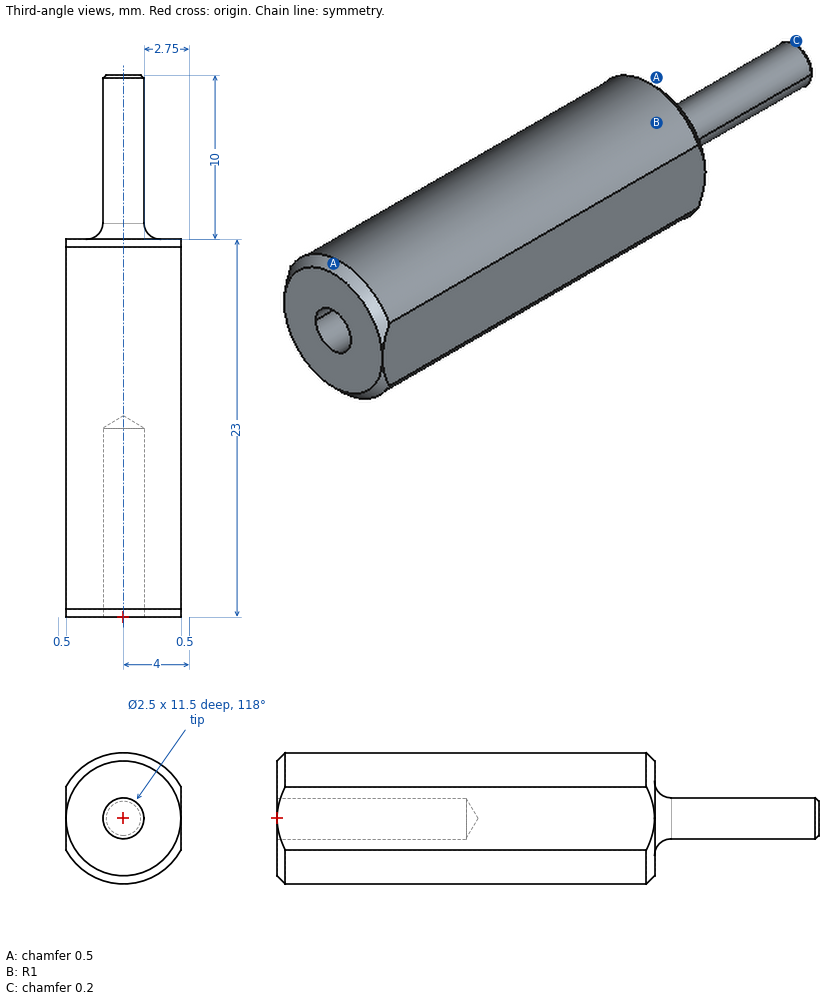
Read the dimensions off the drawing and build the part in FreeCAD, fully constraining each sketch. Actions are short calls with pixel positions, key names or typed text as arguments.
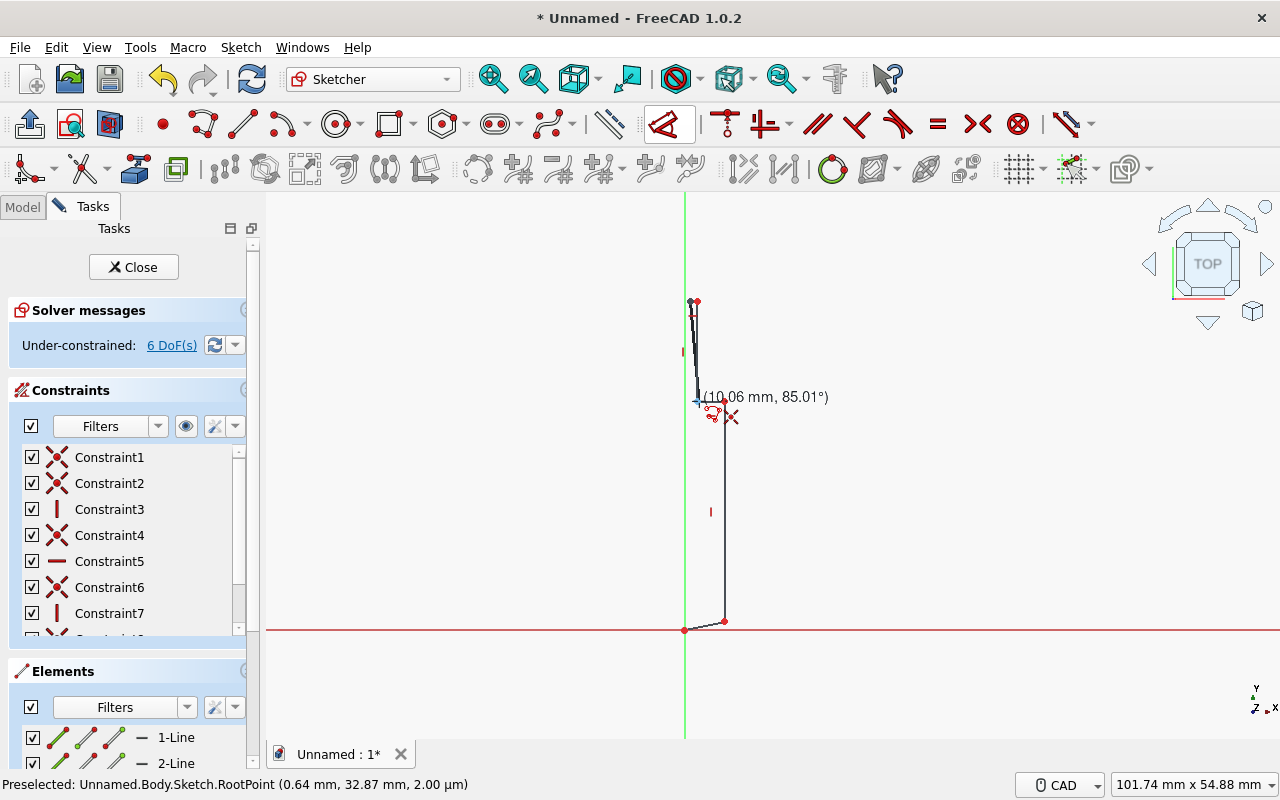
click(685, 630)
key(Escape)
key(Escape)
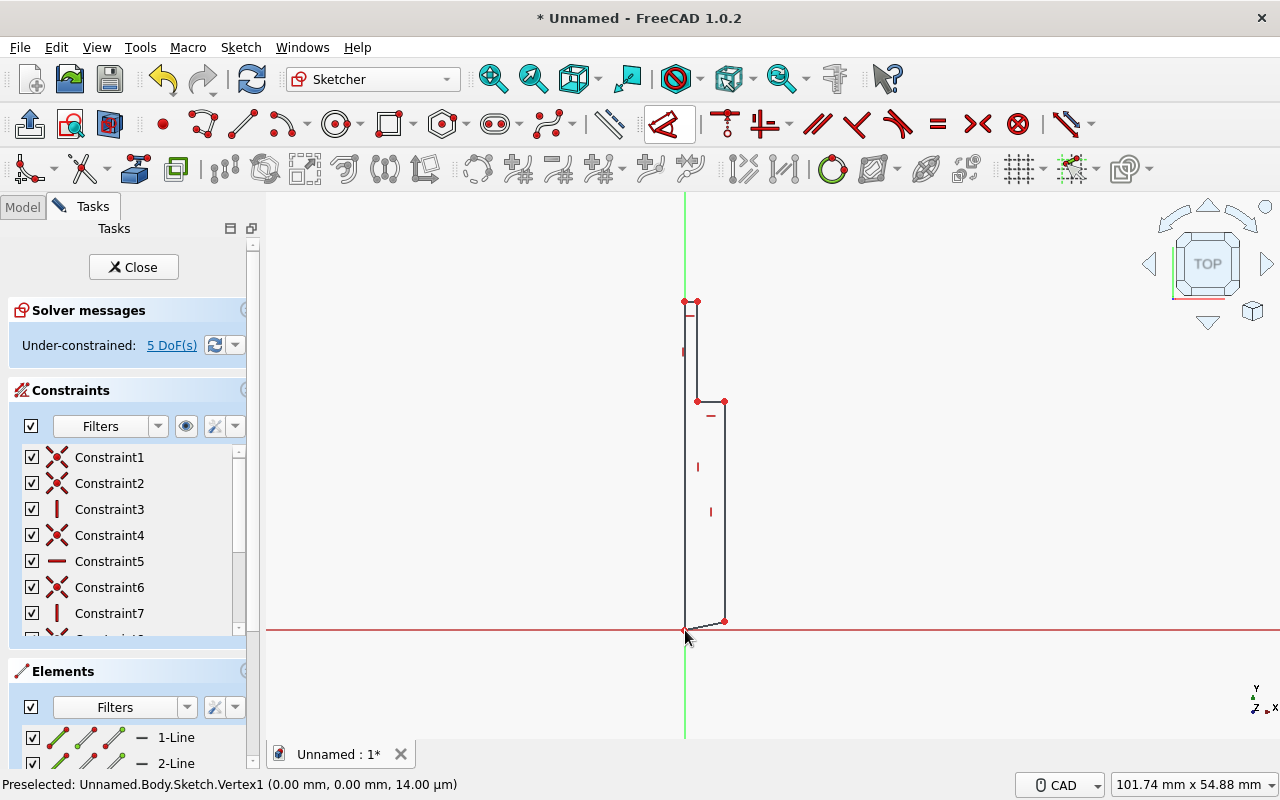
click(697, 628)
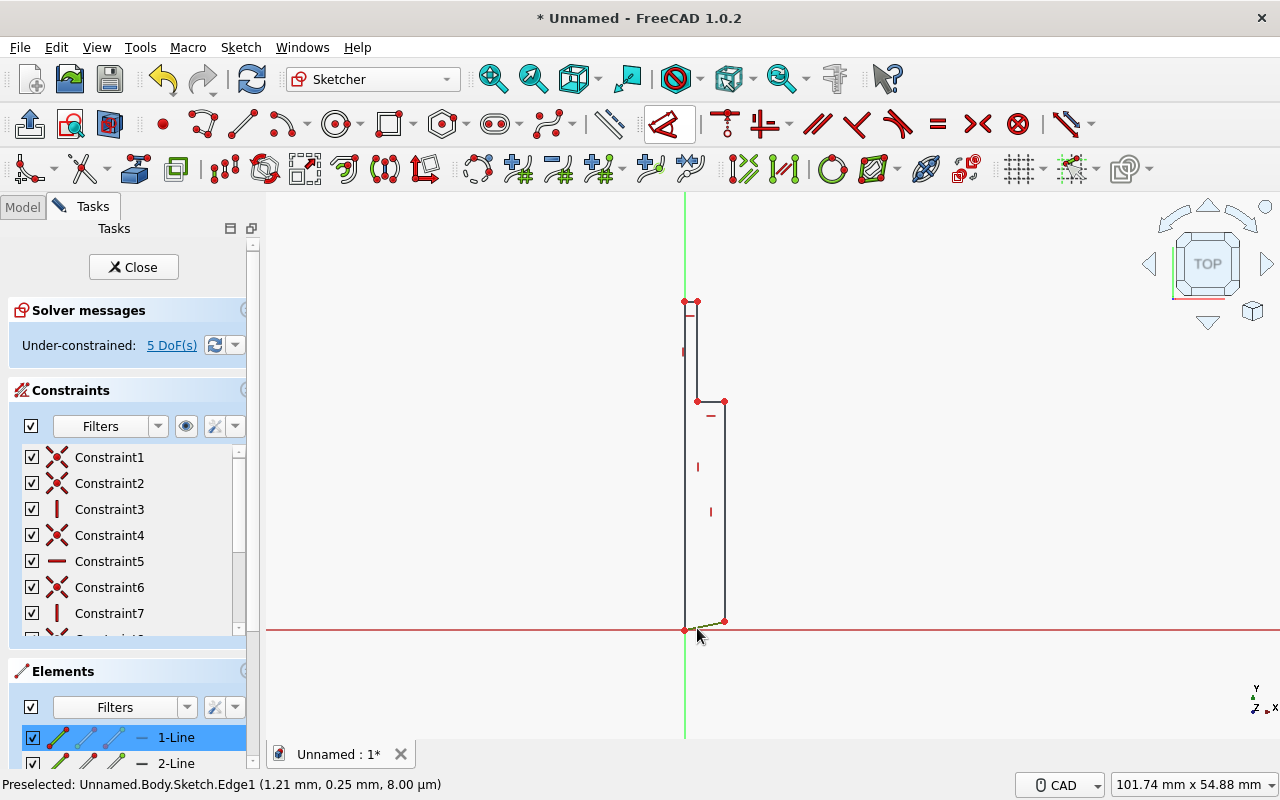
key(h)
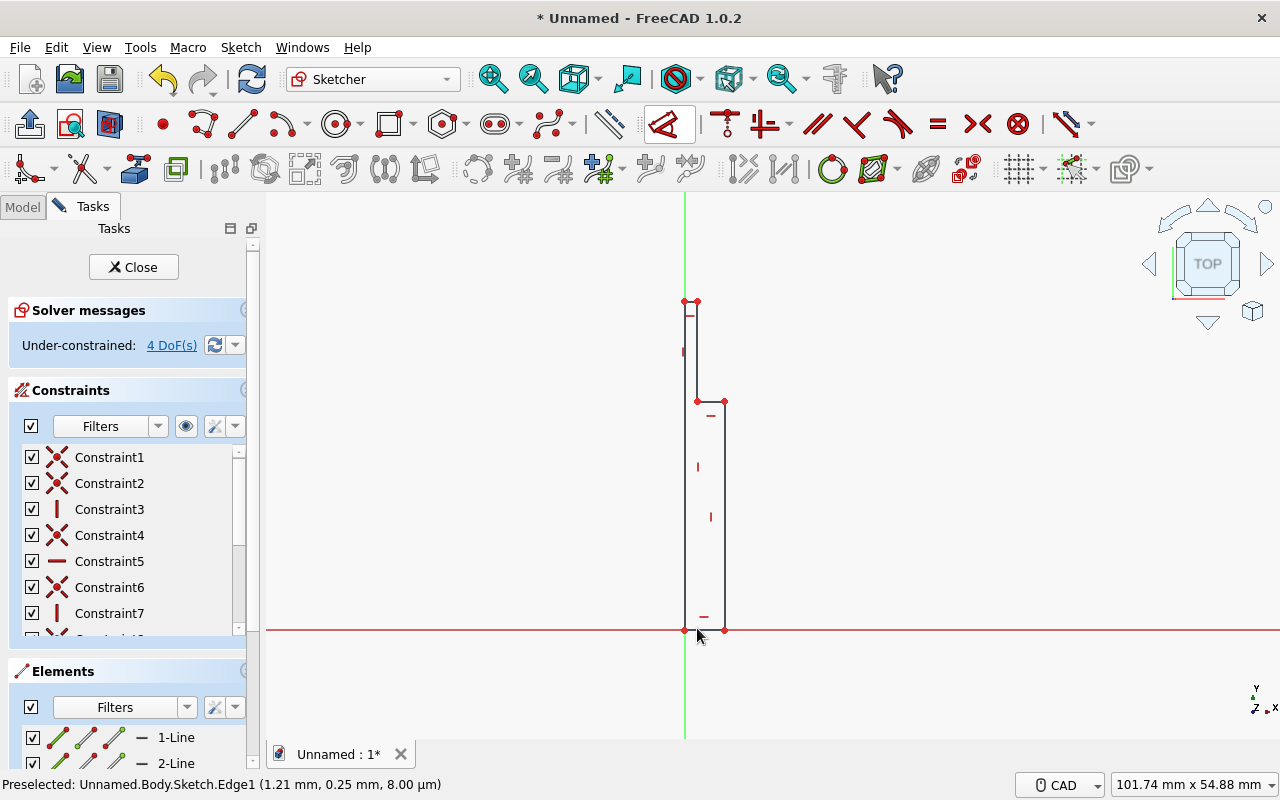
click(697, 630)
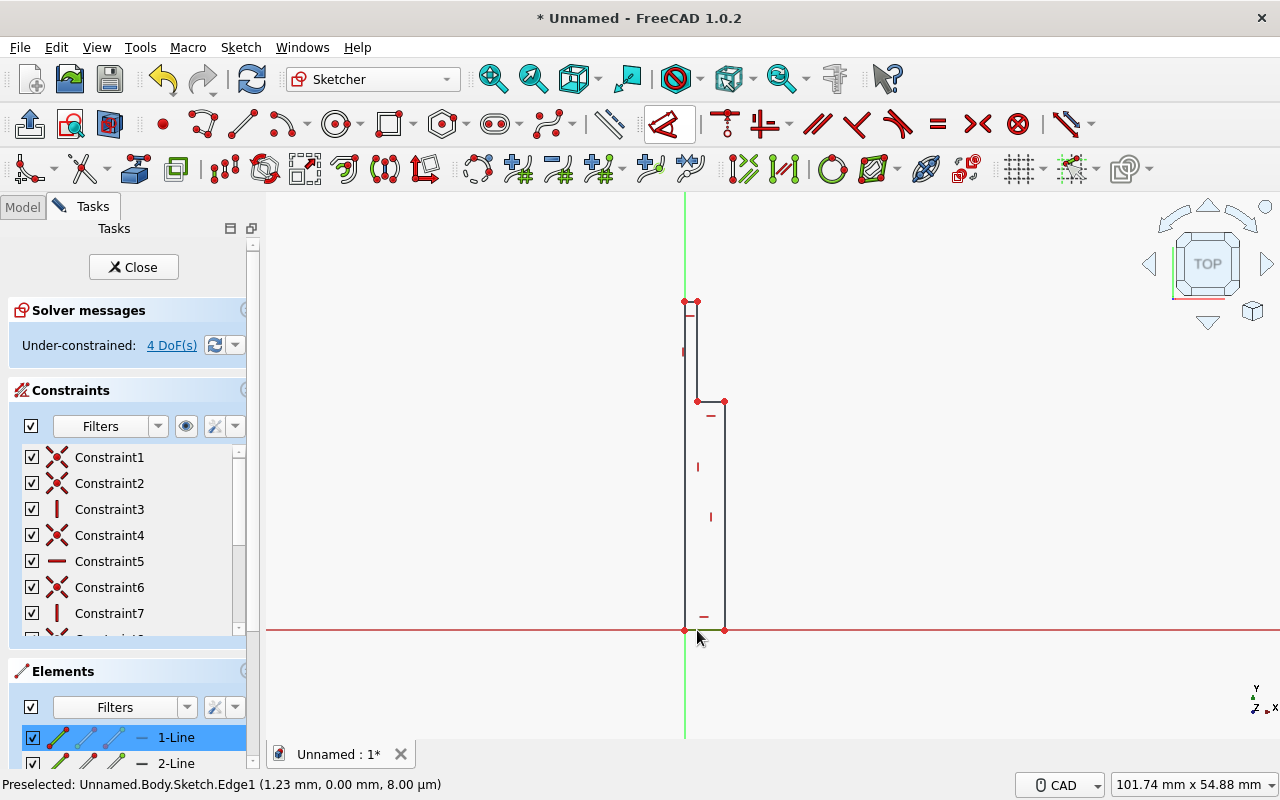
key(l)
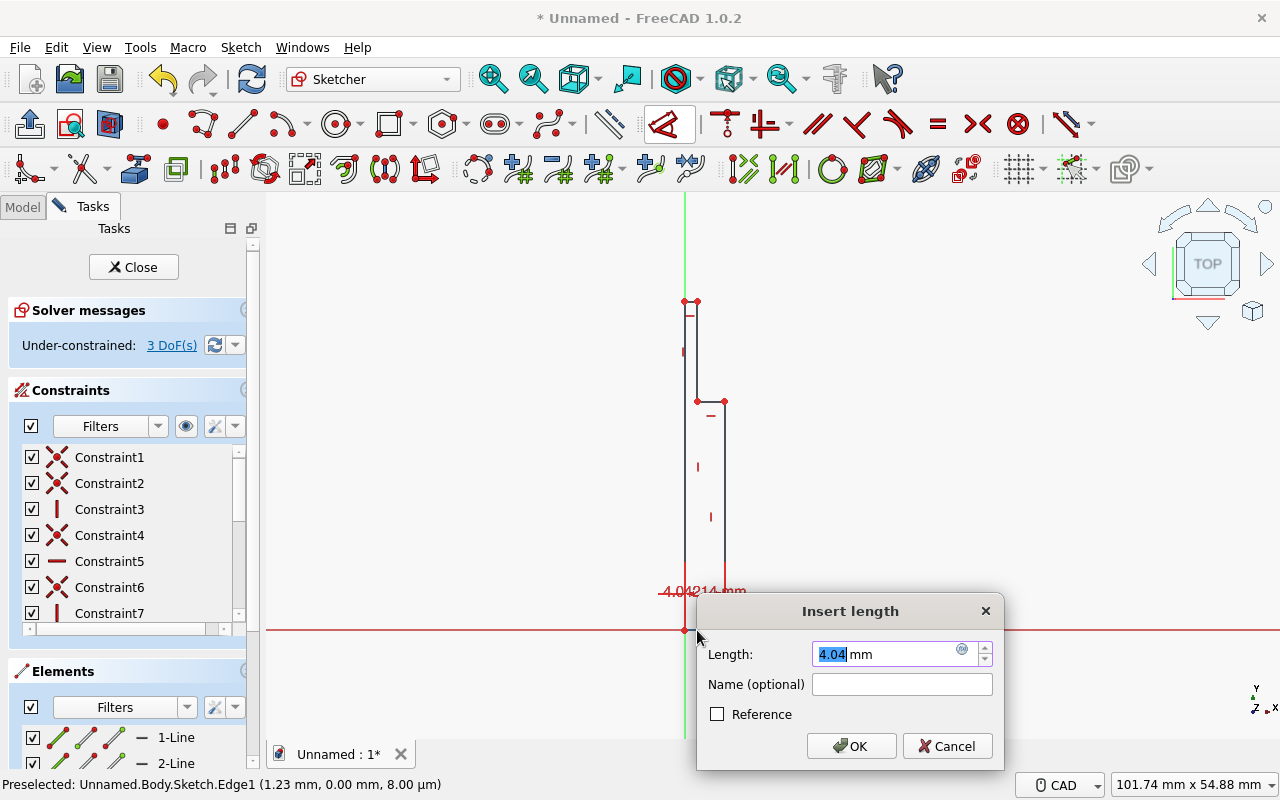
text(4)
key(Return)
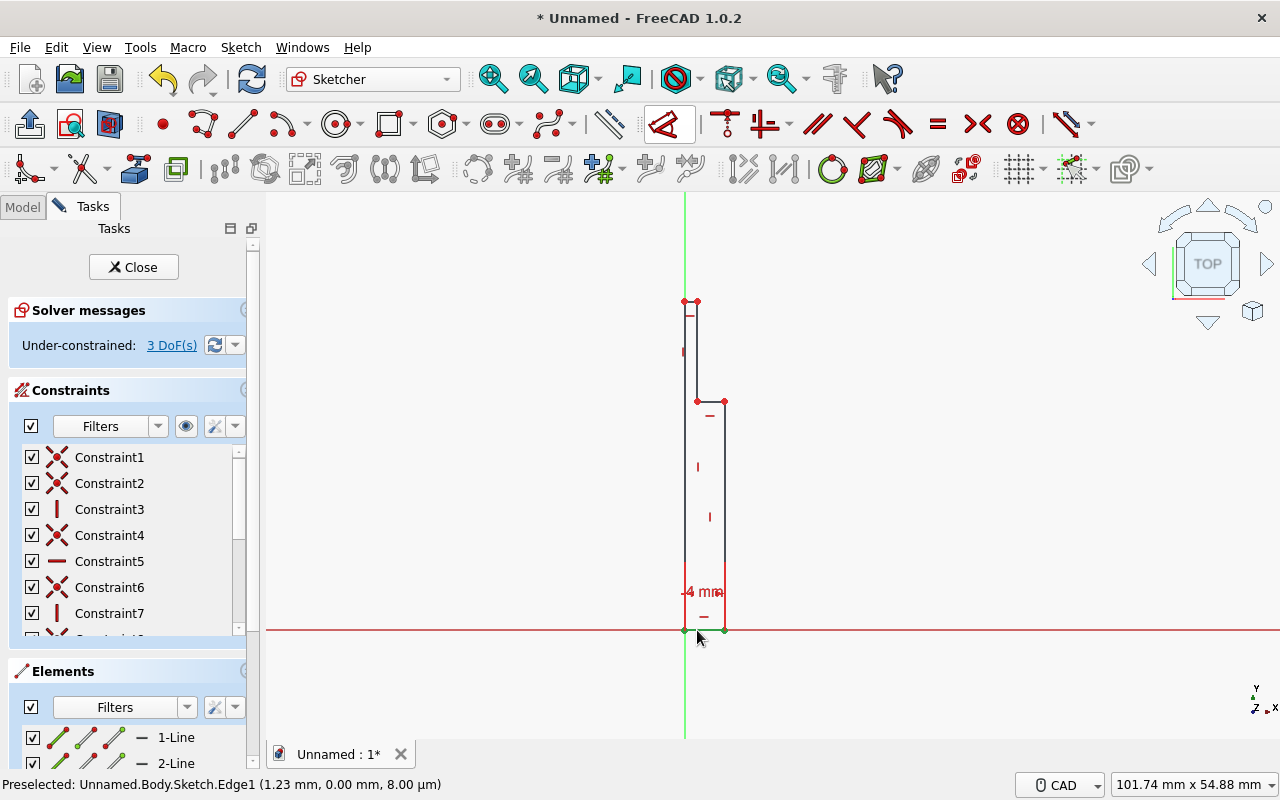
click(725, 562)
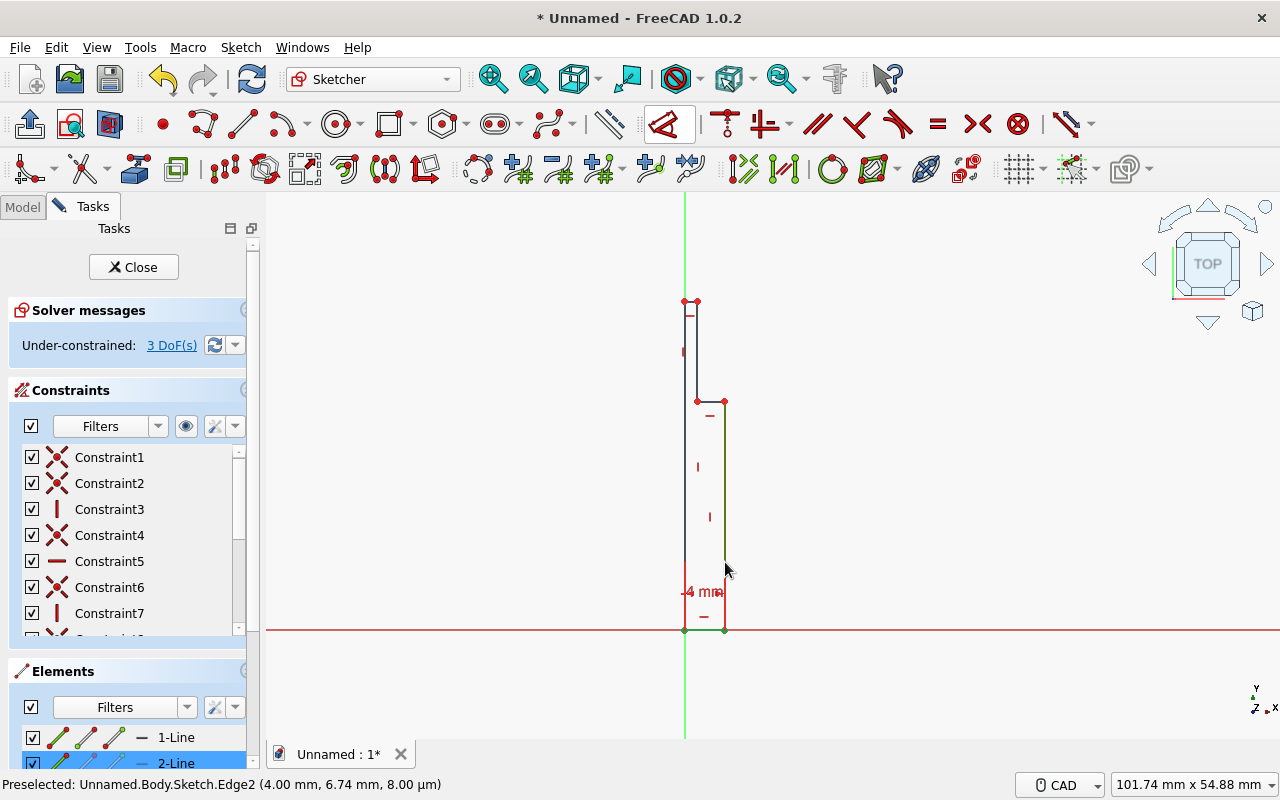
key(i)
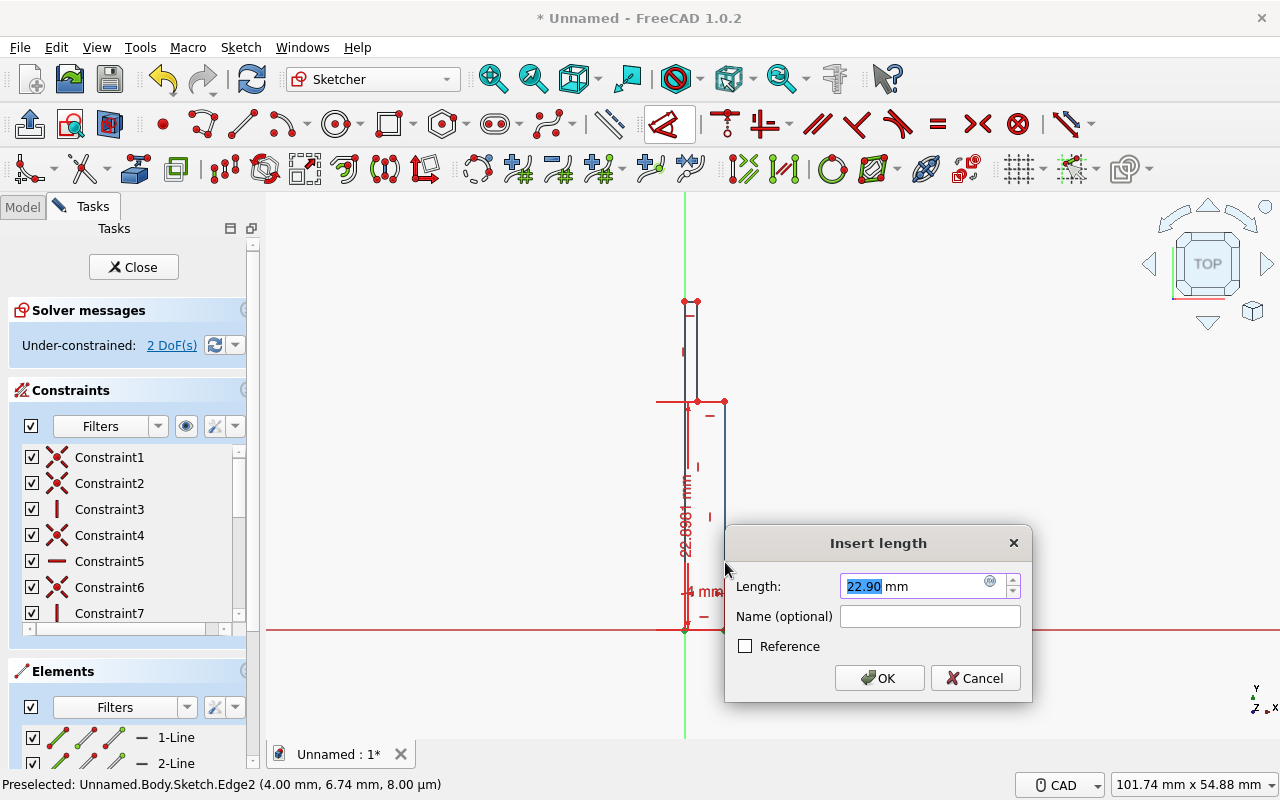
text(23)
key(Return)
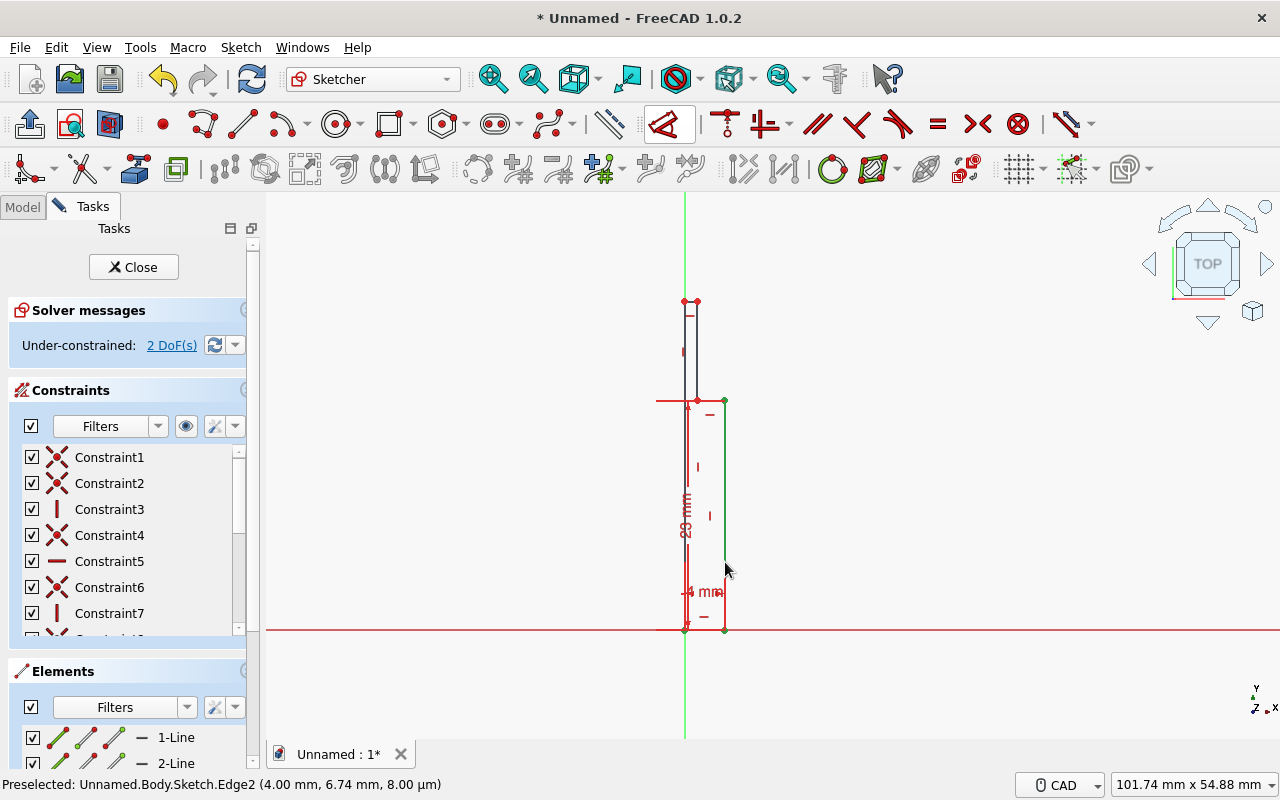
click(697, 371)